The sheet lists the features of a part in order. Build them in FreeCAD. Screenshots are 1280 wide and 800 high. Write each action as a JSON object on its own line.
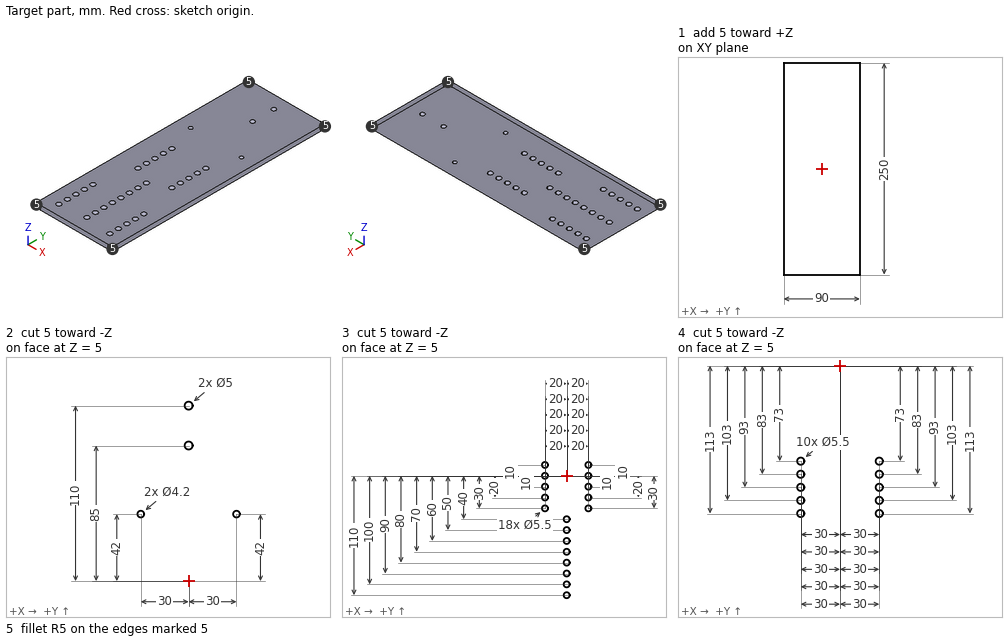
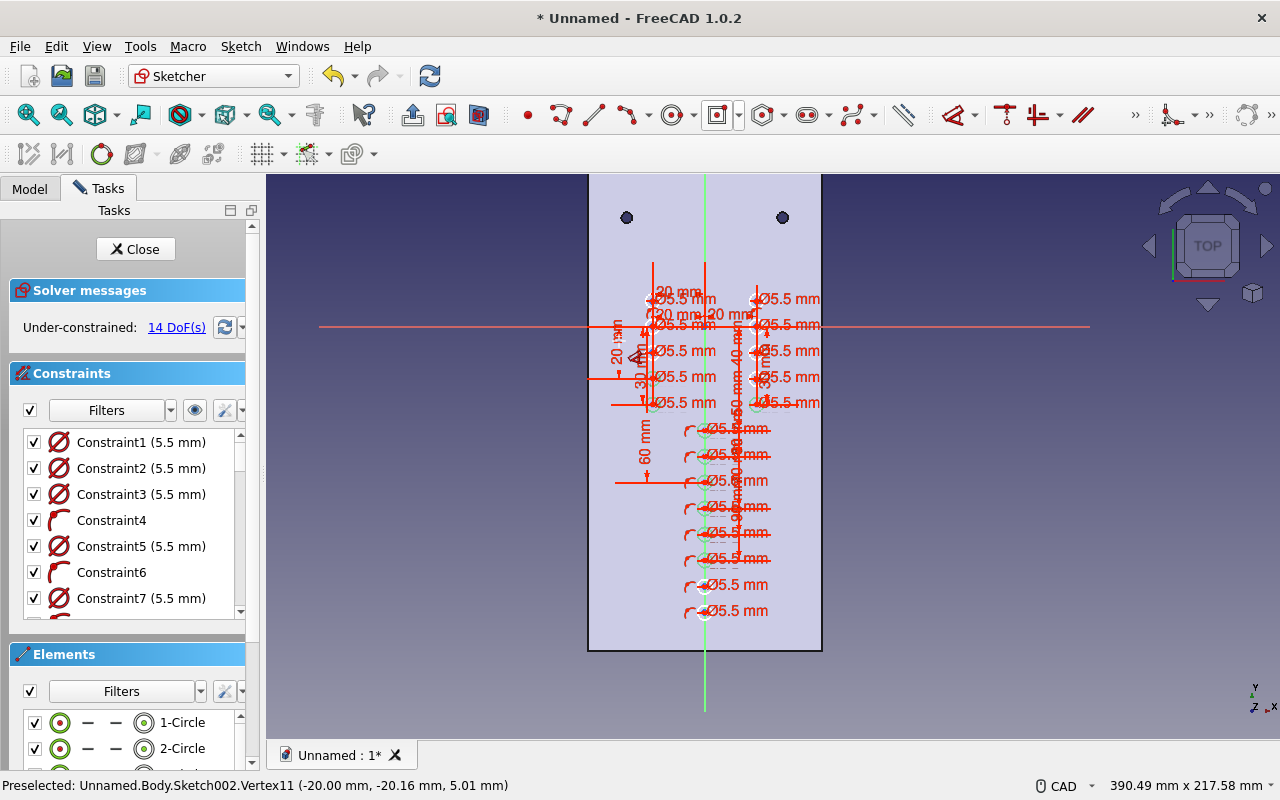
{"action": "left_click", "coordinate": [757, 379]}
{"action": "left_click", "coordinate": [731, 269]}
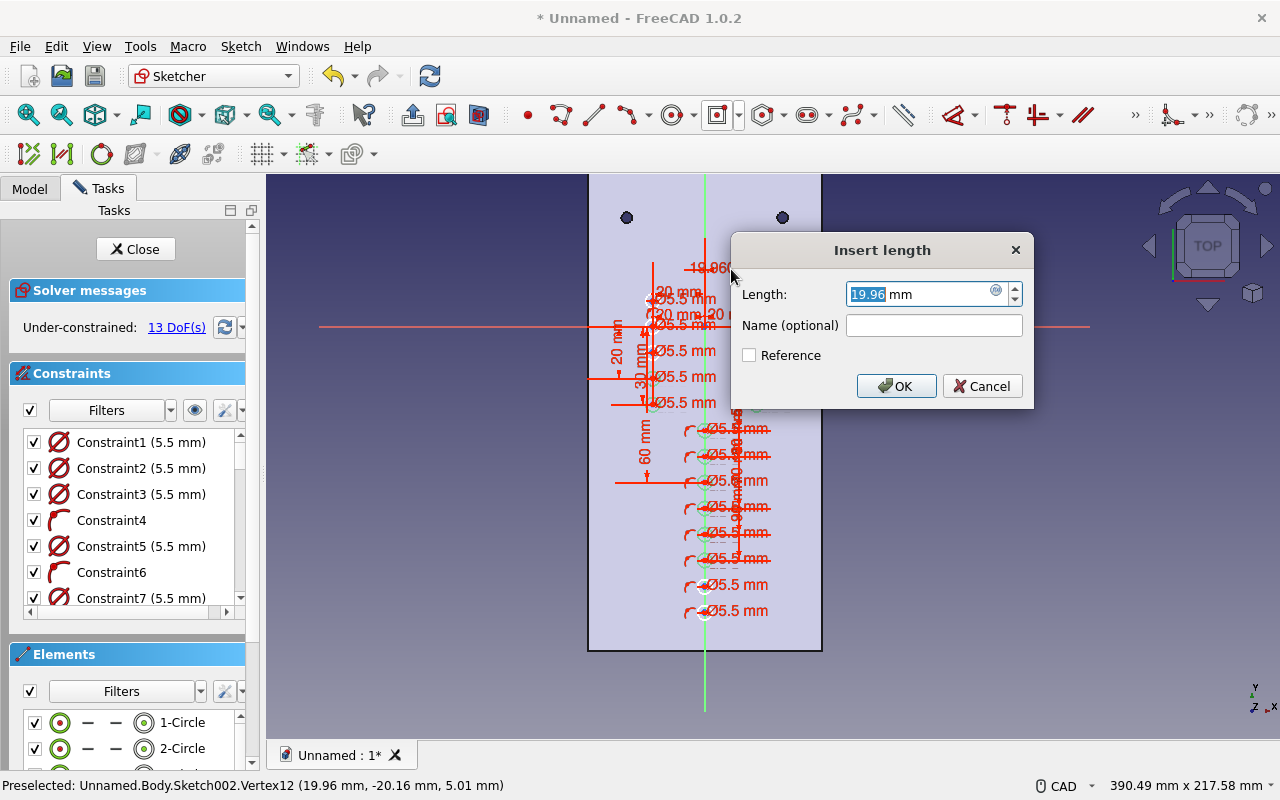
{"action": "type", "text": "20"}
{"action": "key", "text": "Return"}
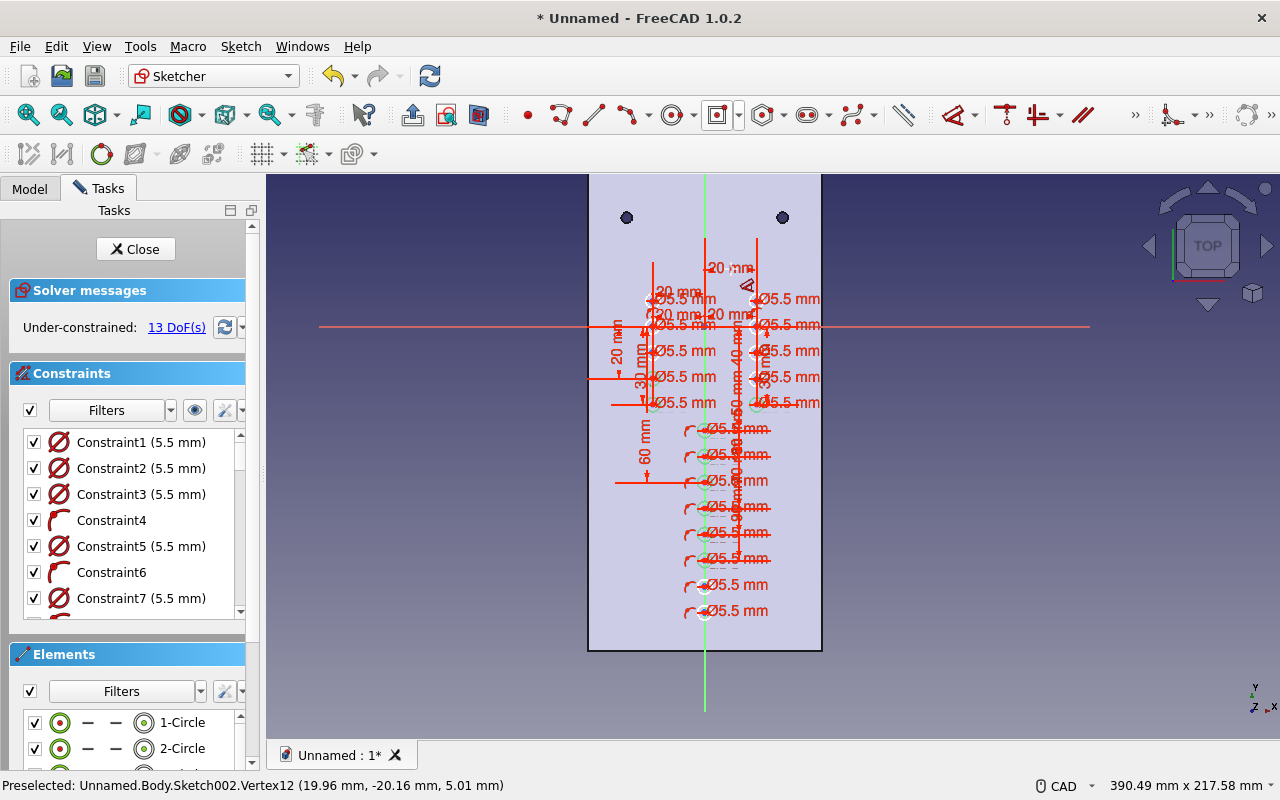
{"action": "left_click", "coordinate": [757, 379]}
{"action": "left_click", "coordinate": [815, 341]}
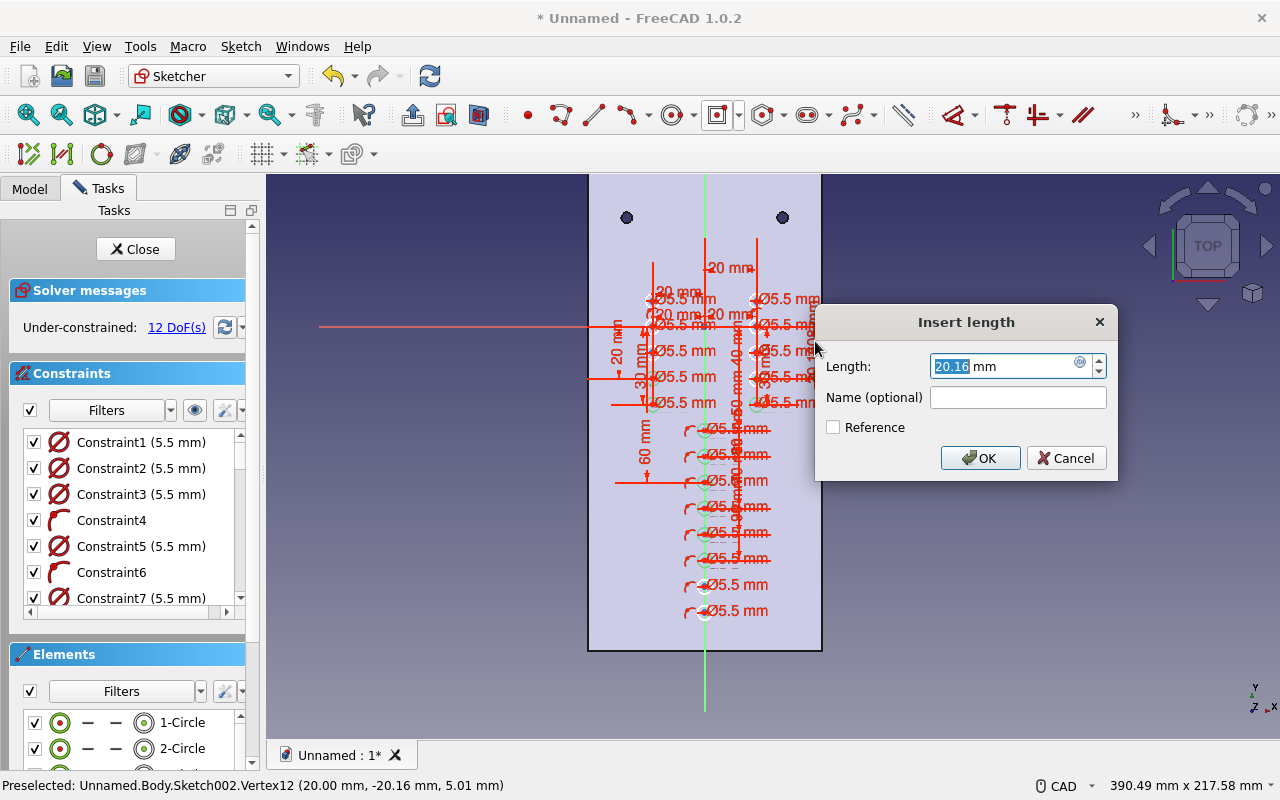
{"action": "type", "text": "20"}
{"action": "key", "text": "Return"}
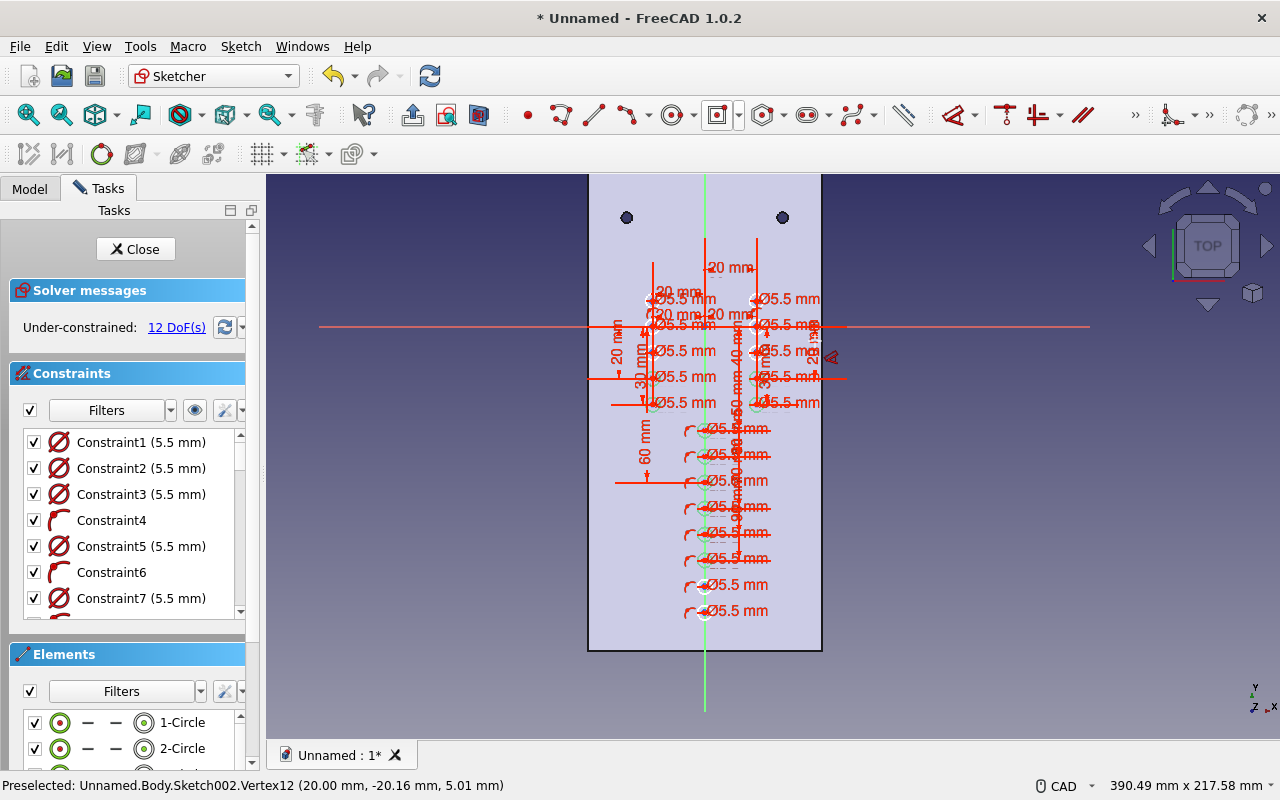
{"action": "left_click", "coordinate": [653, 353]}
{"action": "left_click", "coordinate": [660, 269]}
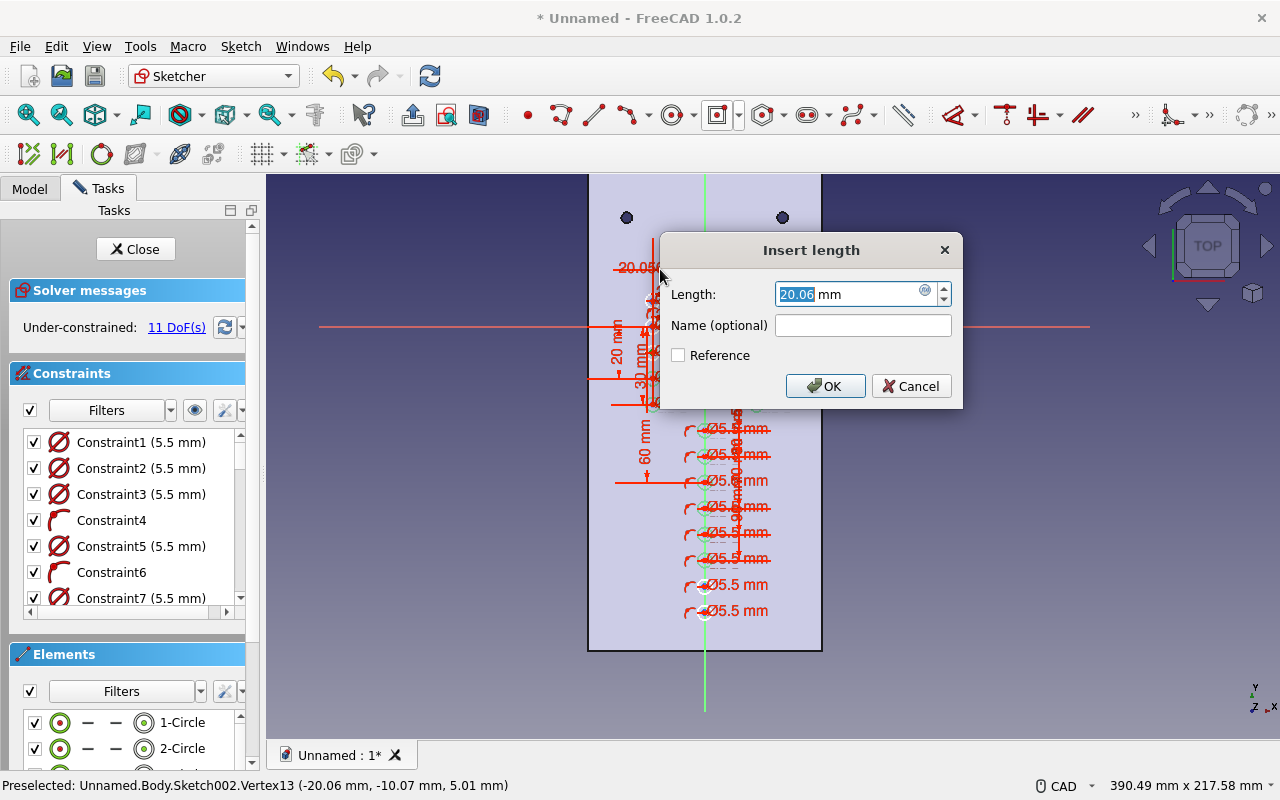
{"action": "type", "text": "20"}
{"action": "key", "text": "Return"}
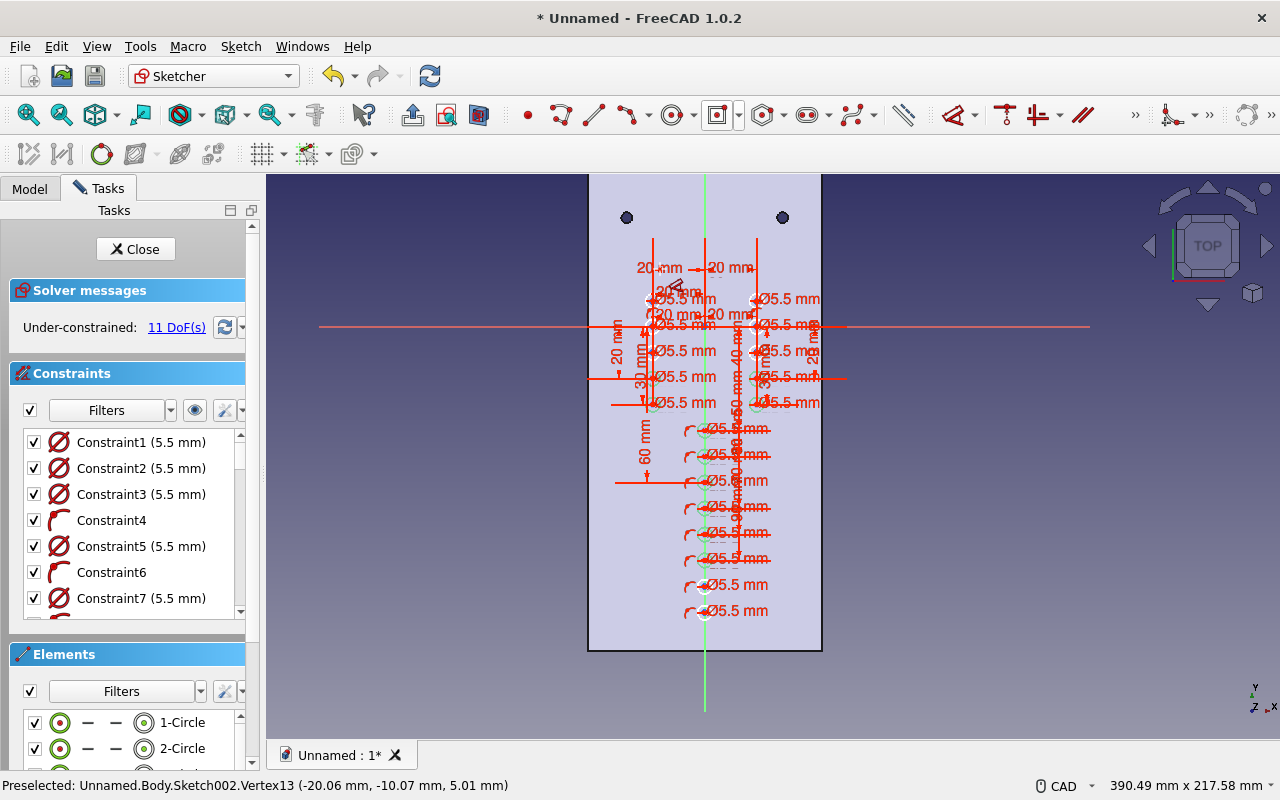
{"action": "scroll", "coordinate": [653, 353], "scroll_direction": "up", "scroll_amount": 3}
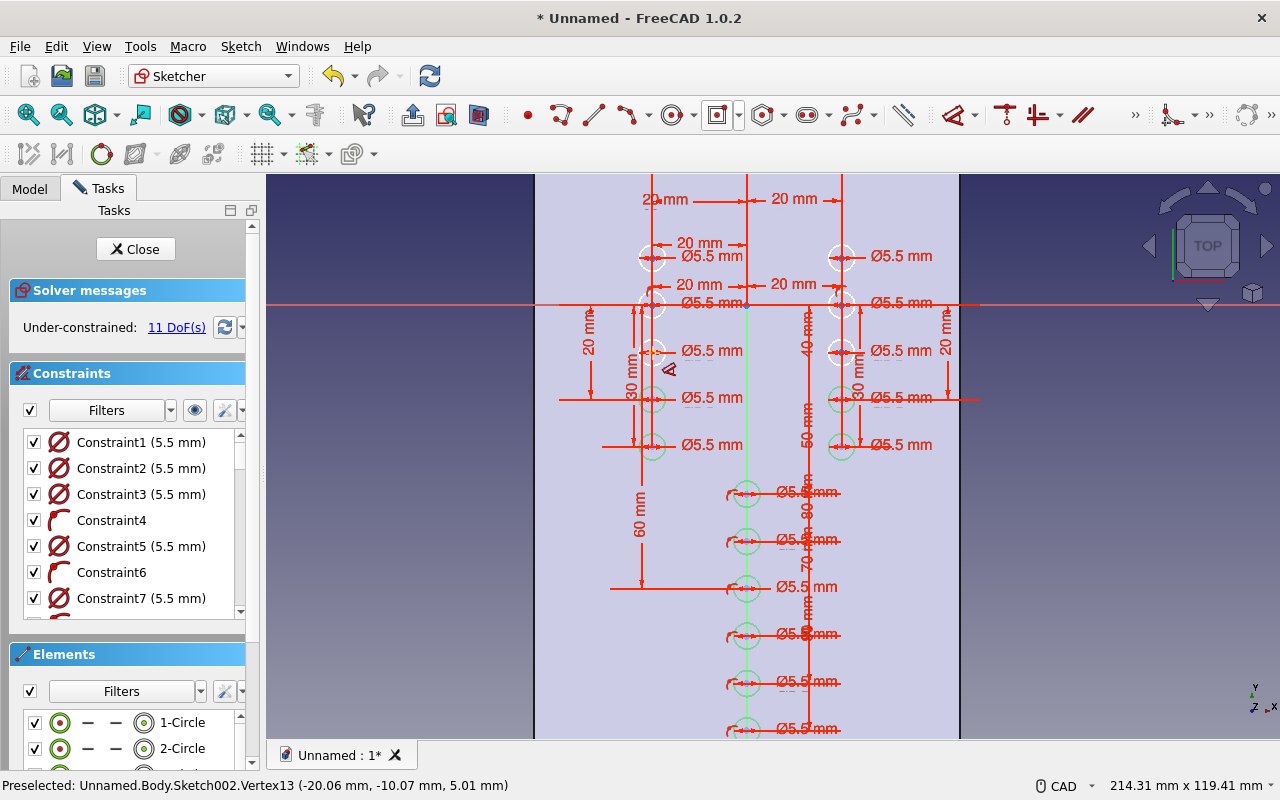
{"action": "left_click", "coordinate": [652, 353]}
{"action": "left_click", "coordinate": [498, 329]}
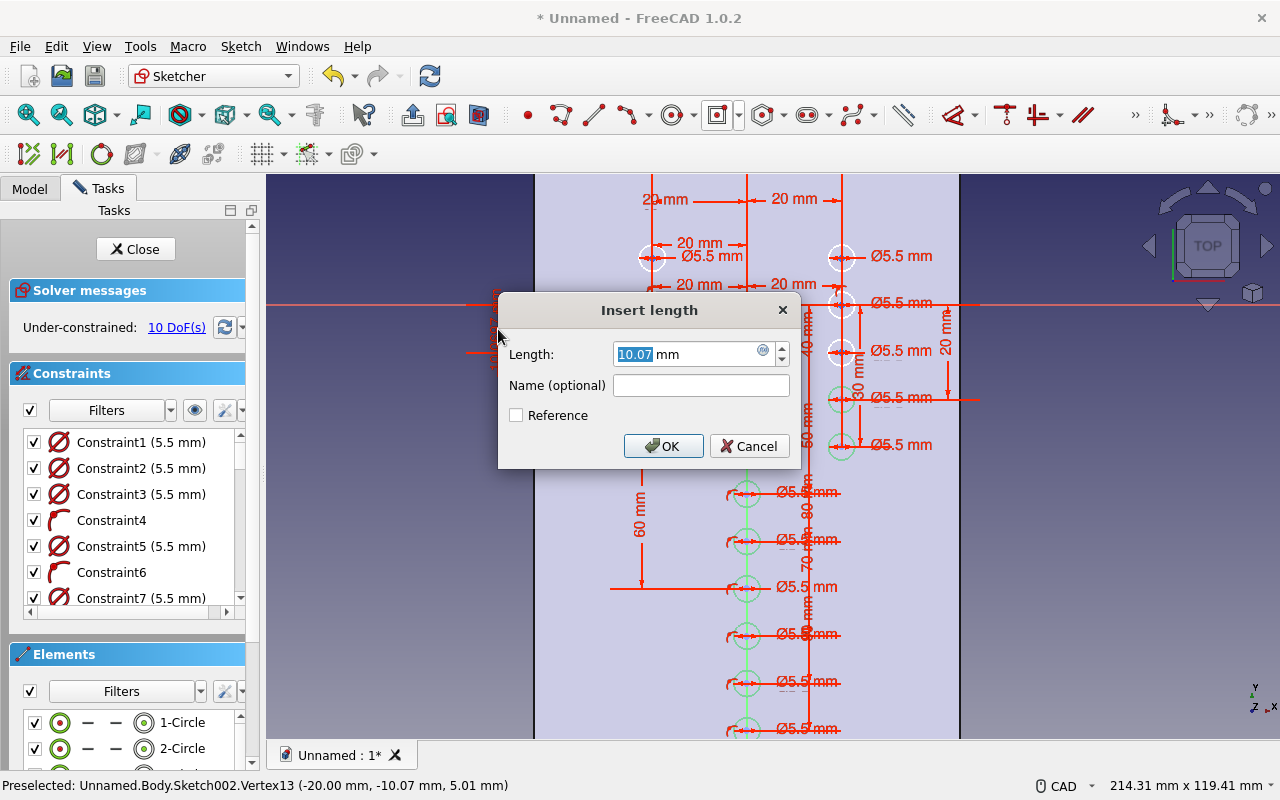
{"action": "type", "text": "10"}
{"action": "key", "text": "Return"}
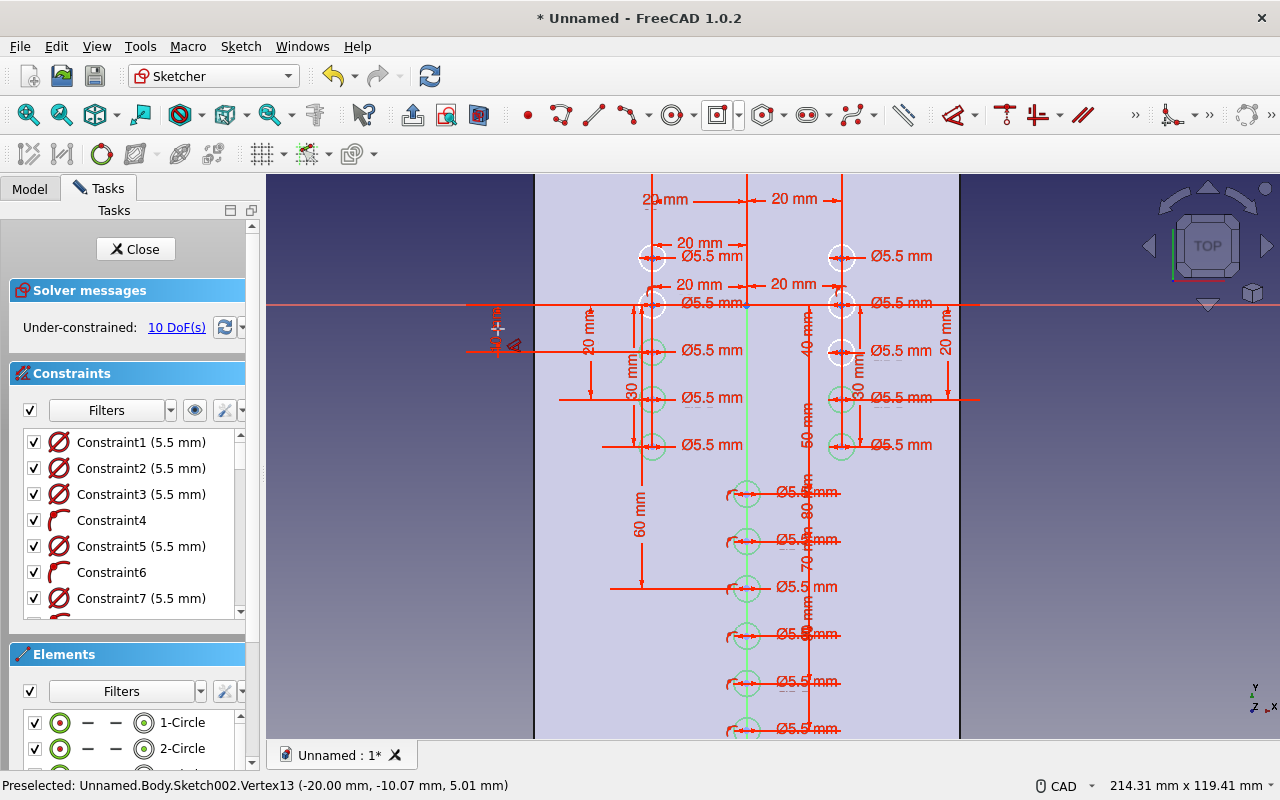
{"action": "left_click", "coordinate": [841, 353]}
{"action": "left_click", "coordinate": [772, 387]}